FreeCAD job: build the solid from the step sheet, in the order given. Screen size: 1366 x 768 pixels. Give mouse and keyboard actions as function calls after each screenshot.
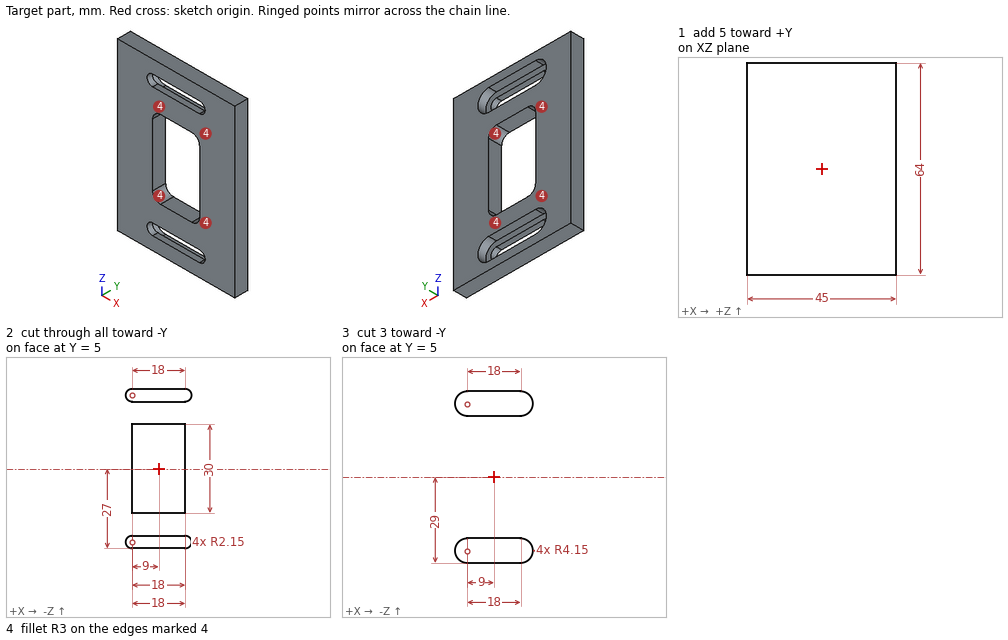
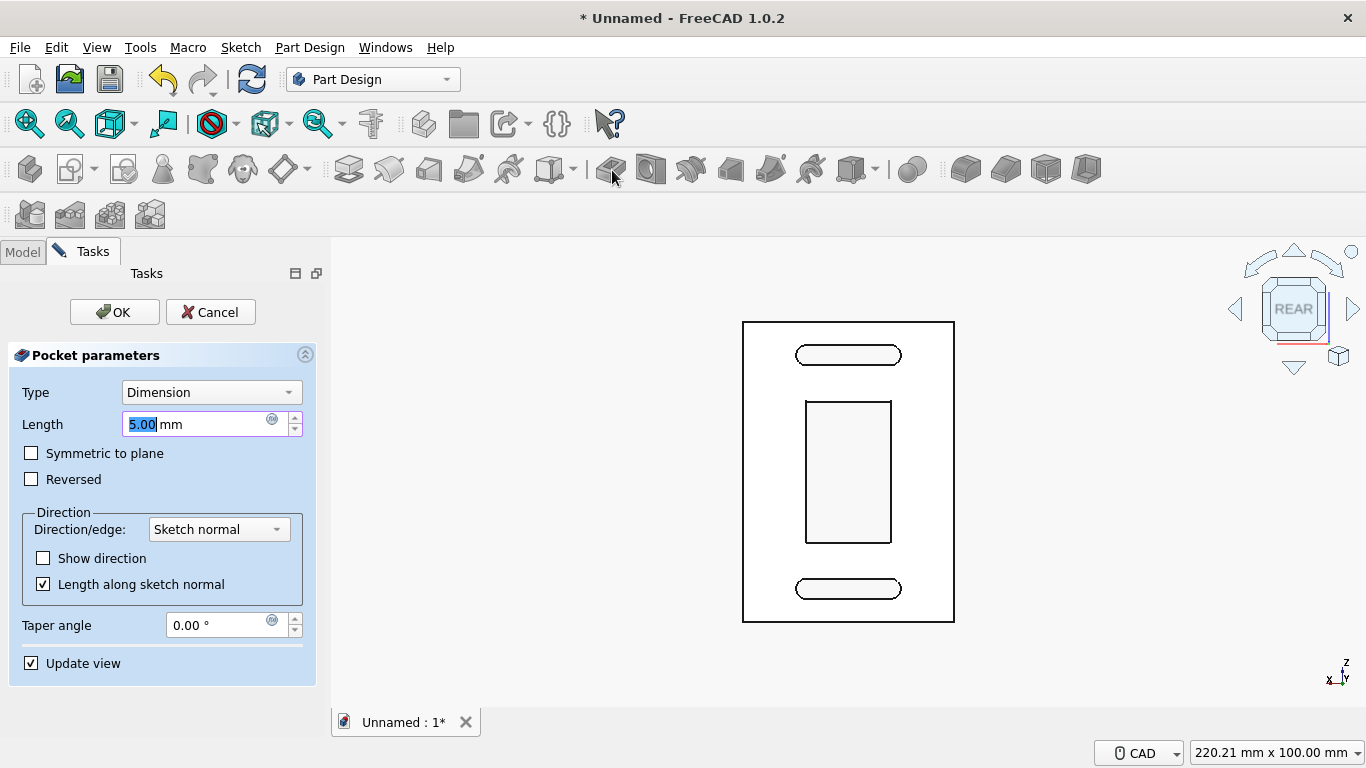
click(212, 392)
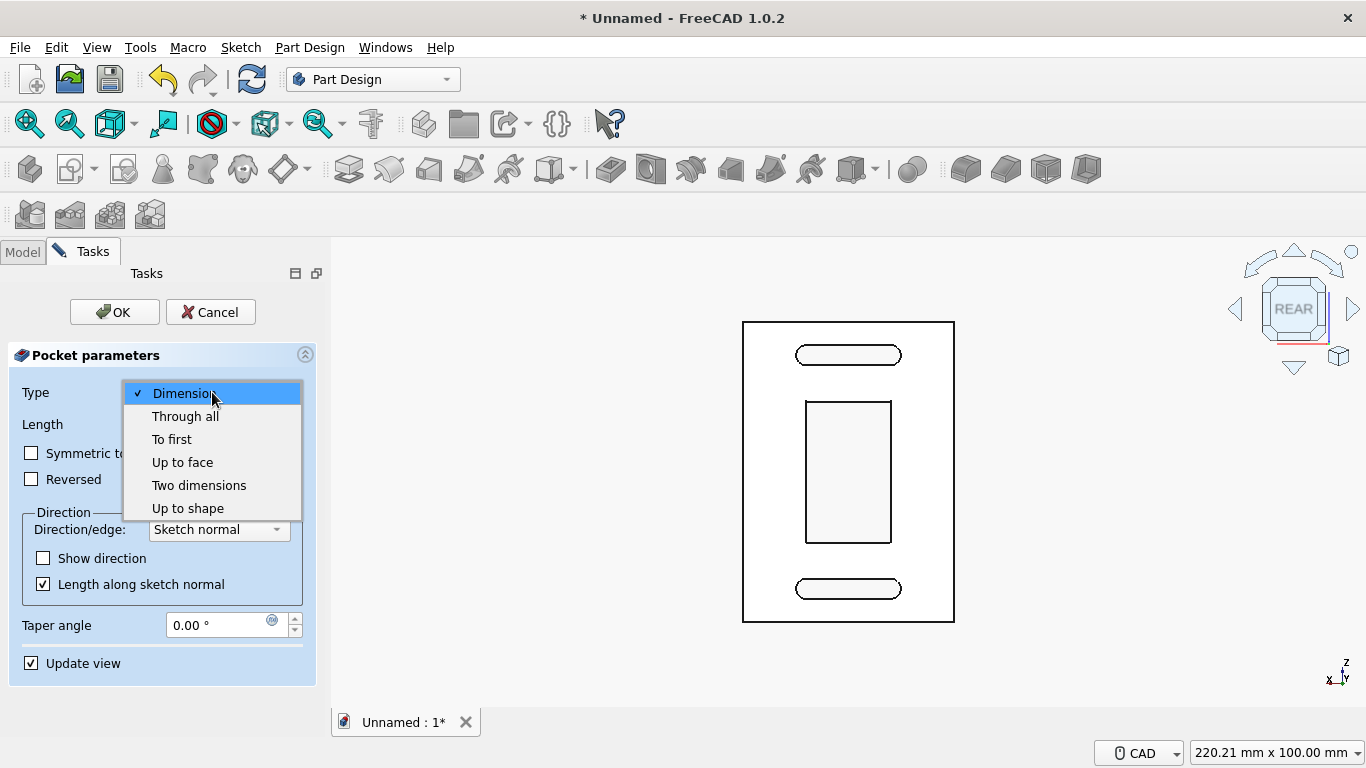
click(212, 416)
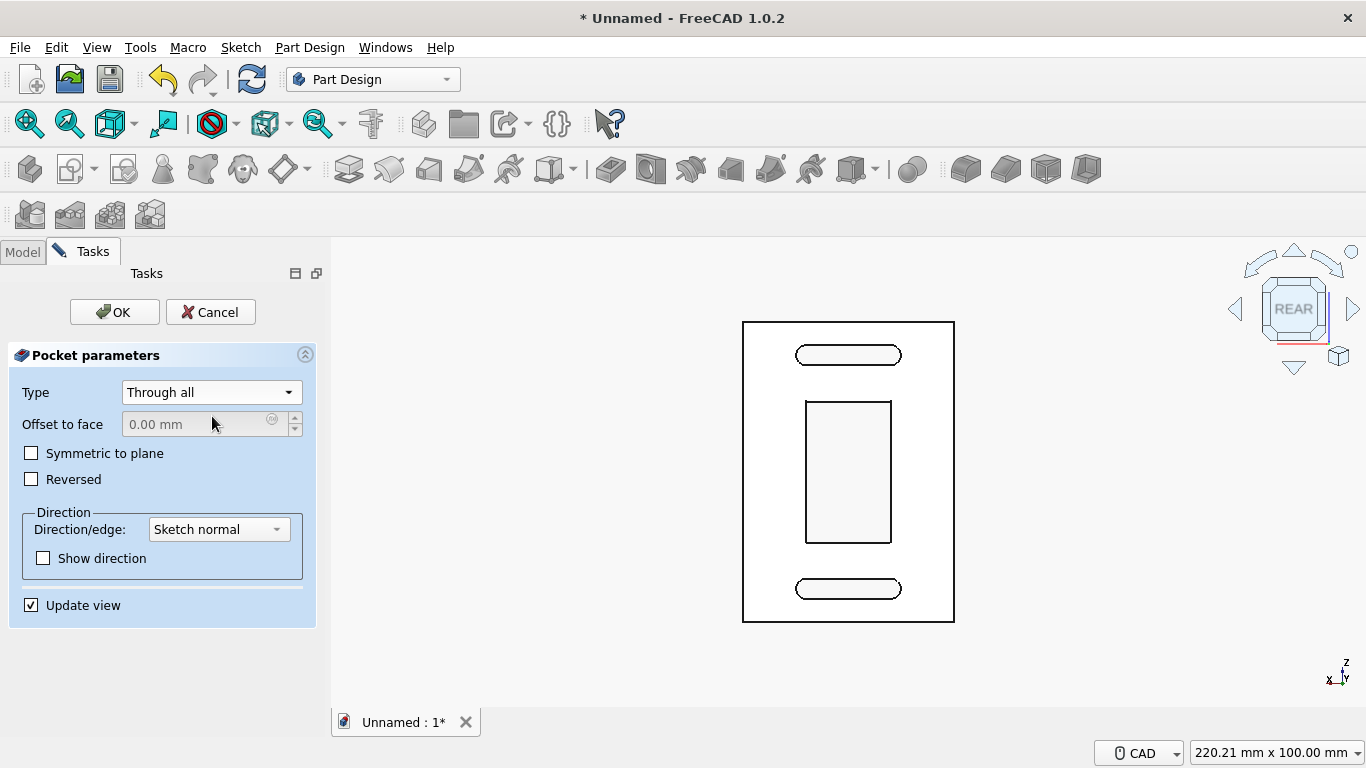
click(115, 312)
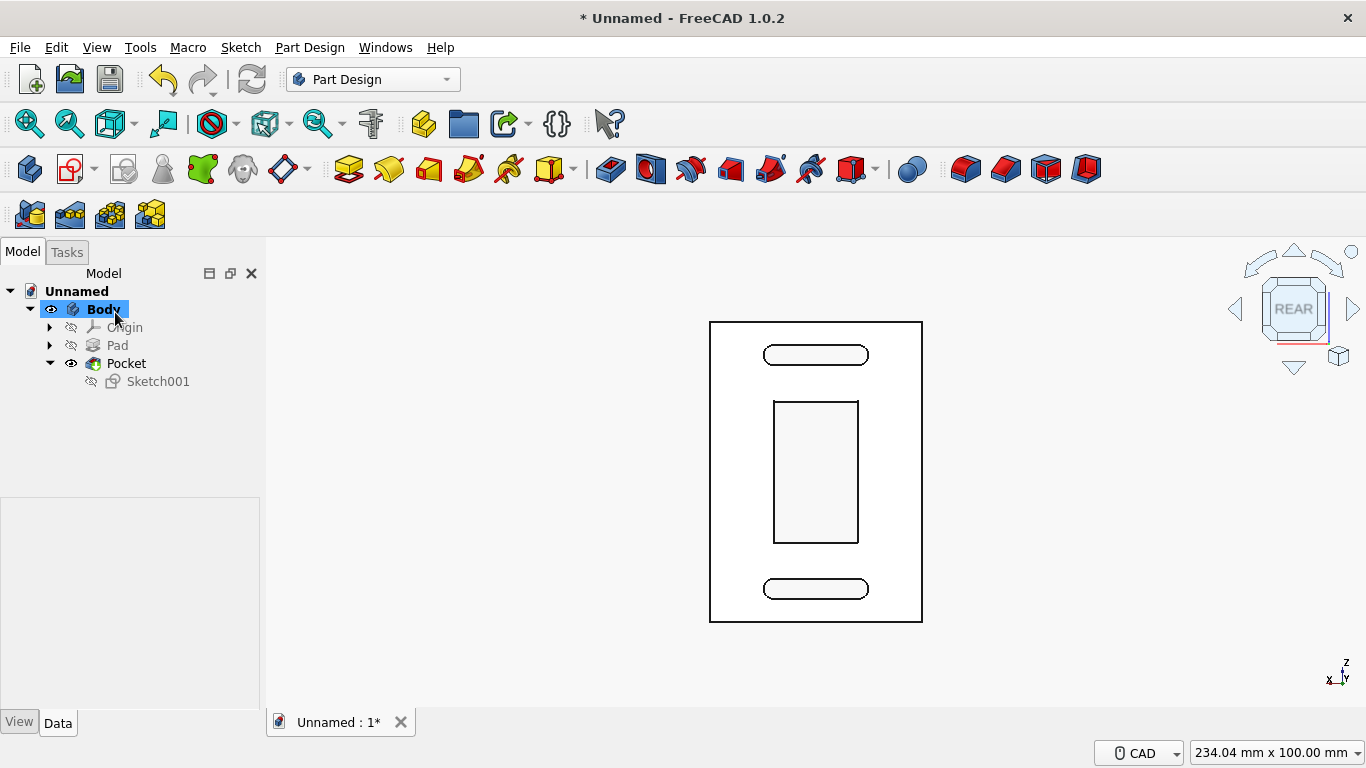
click(876, 385)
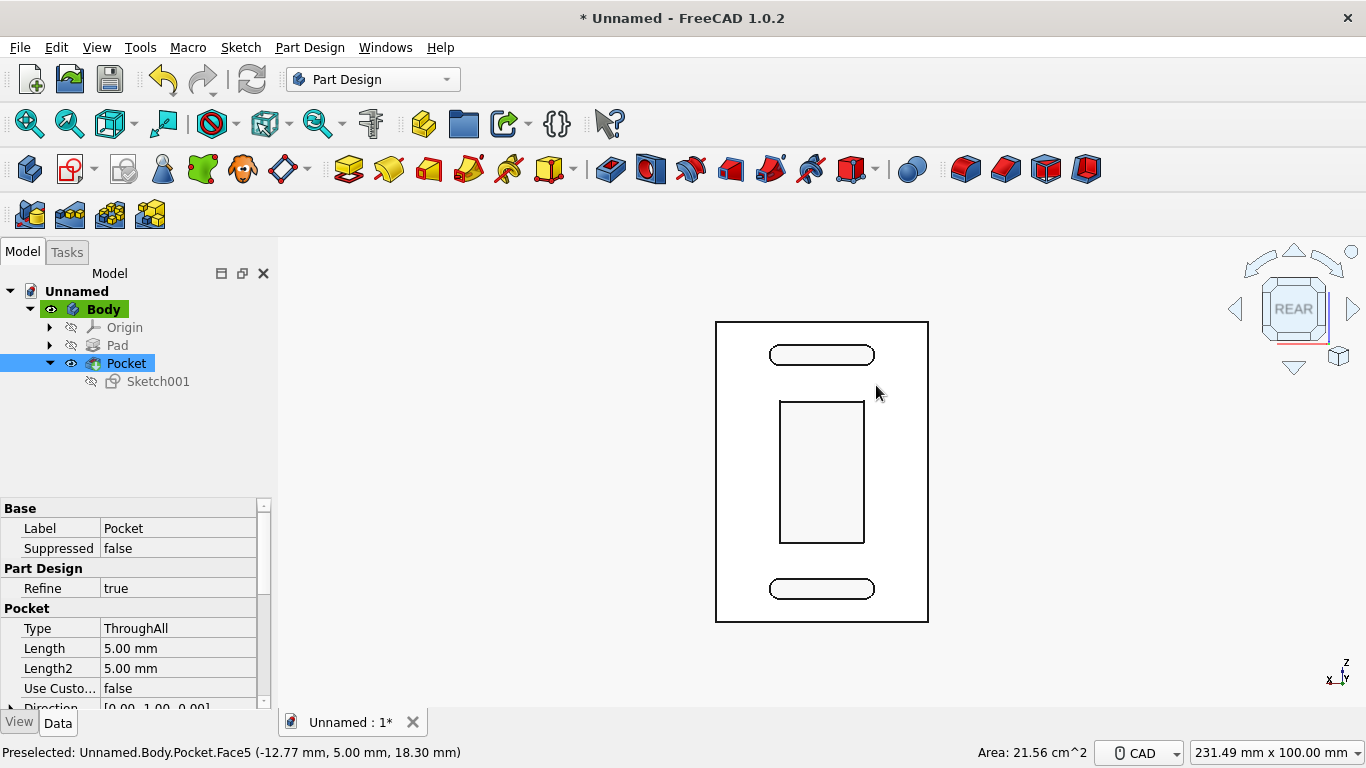
click(70, 170)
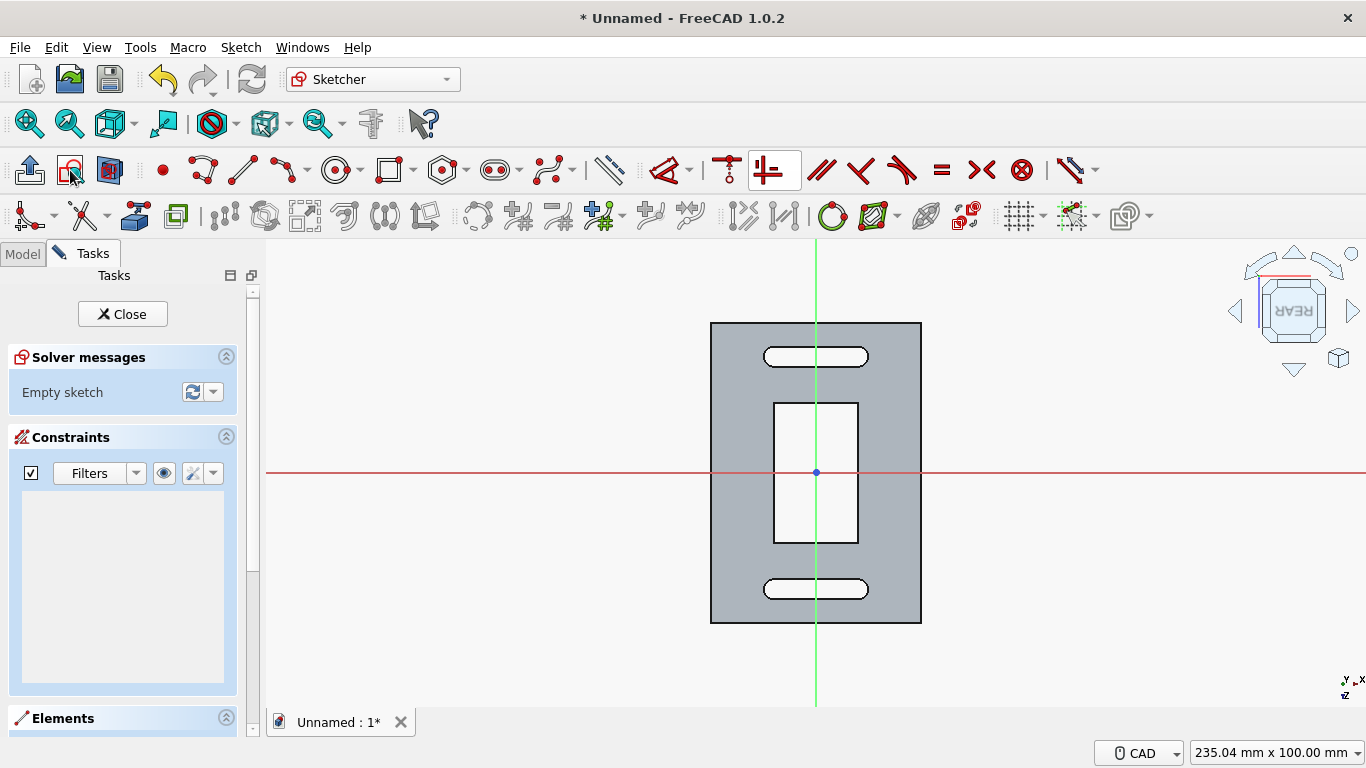
click(496, 170)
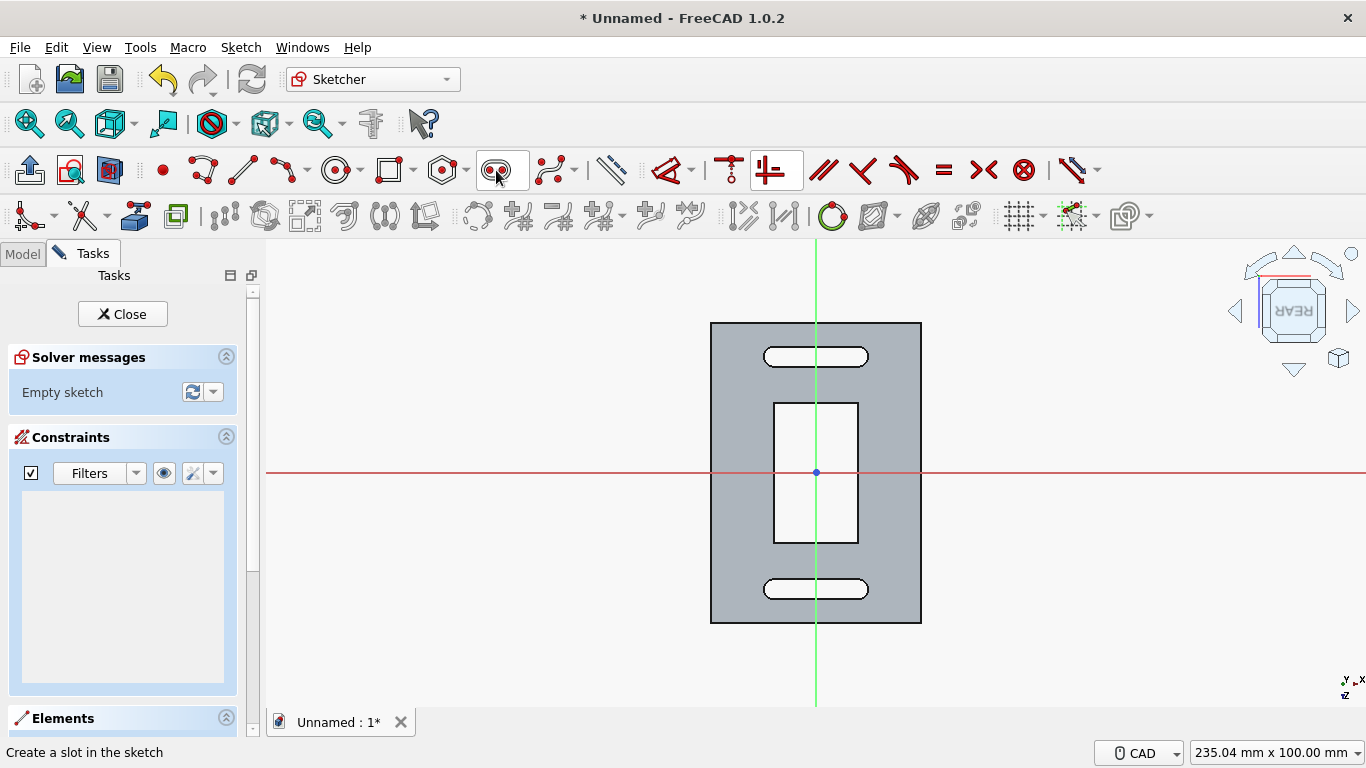
click(774, 589)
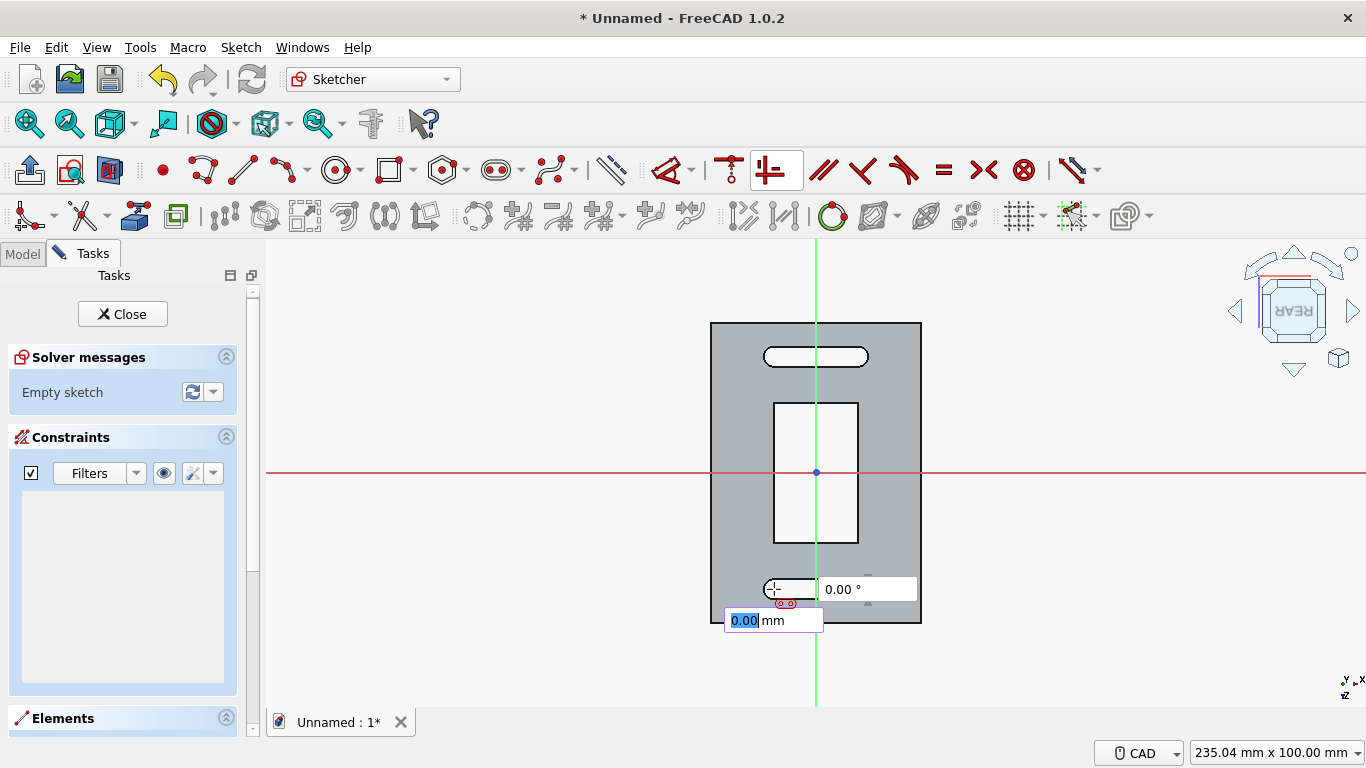
click(858, 589)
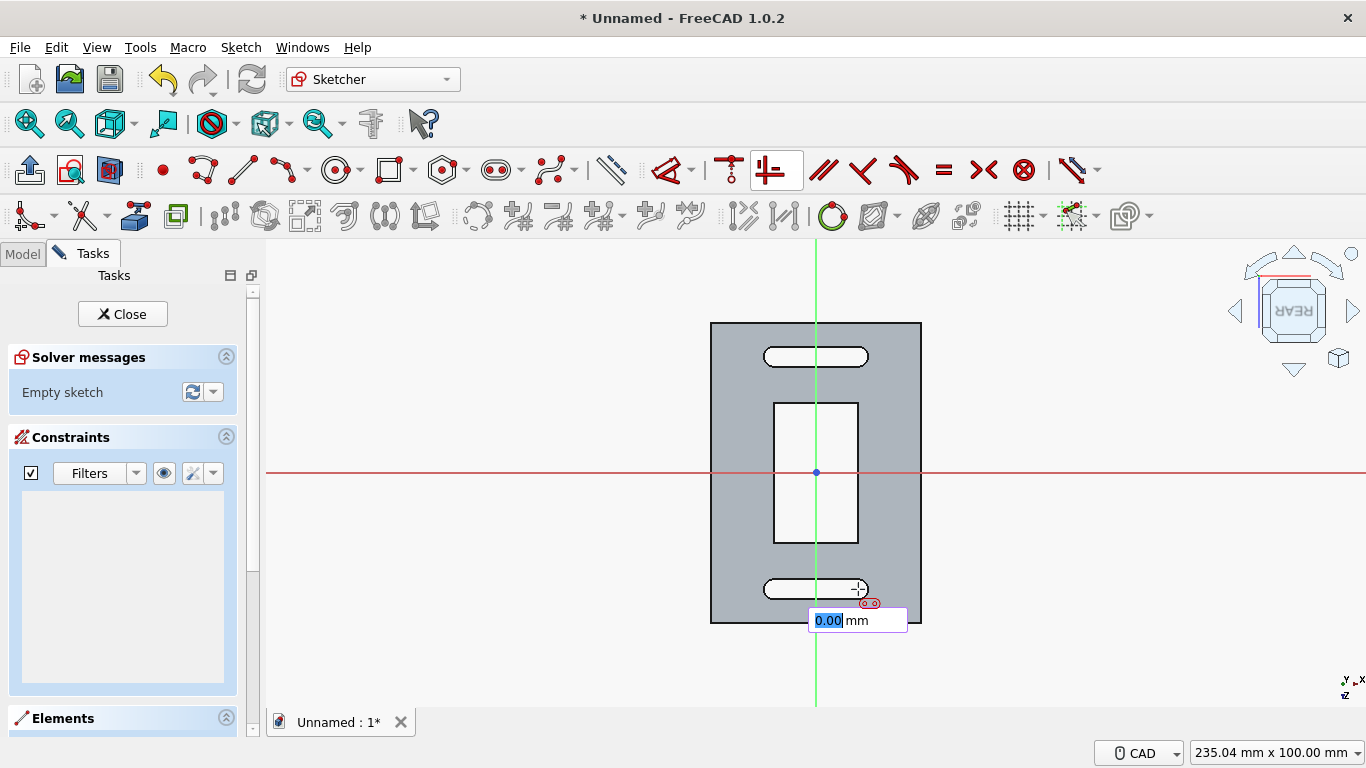
scroll(803, 570, up, 2)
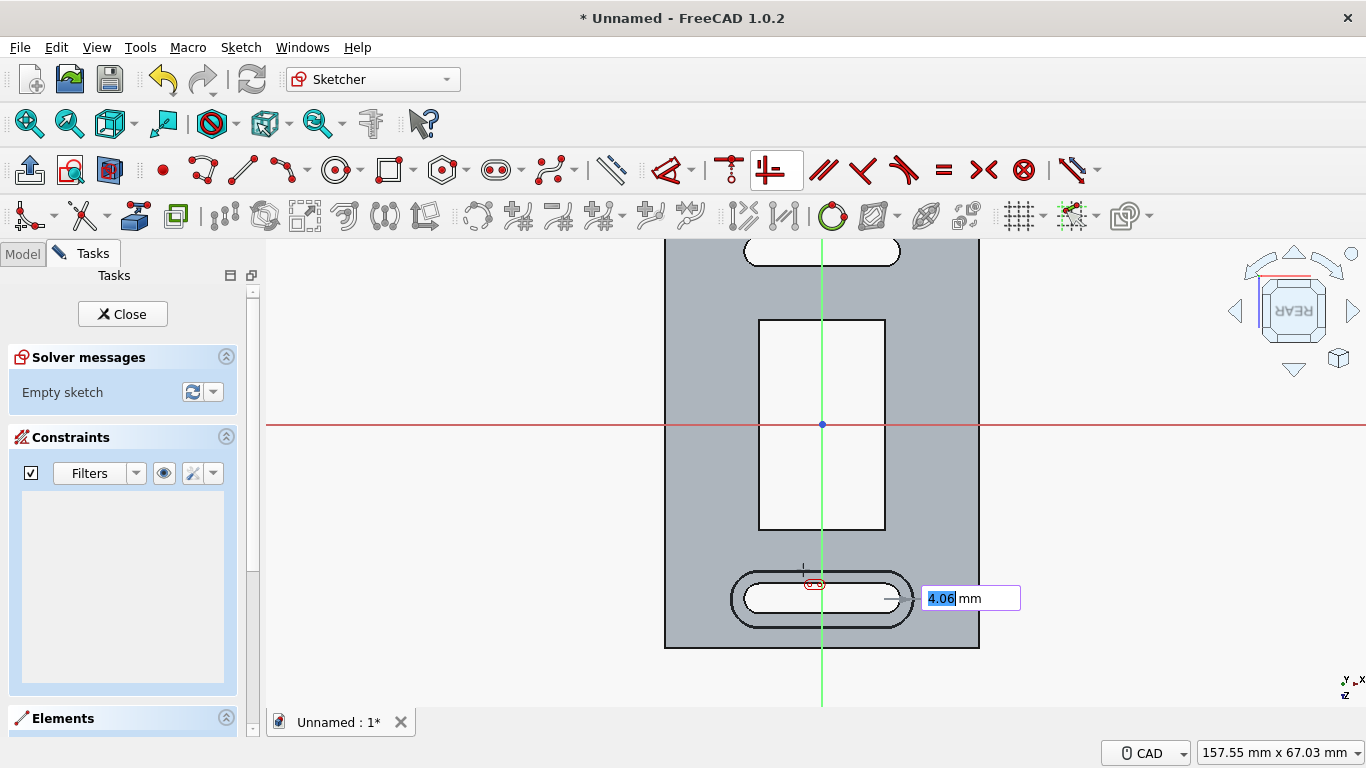
click(803, 569)